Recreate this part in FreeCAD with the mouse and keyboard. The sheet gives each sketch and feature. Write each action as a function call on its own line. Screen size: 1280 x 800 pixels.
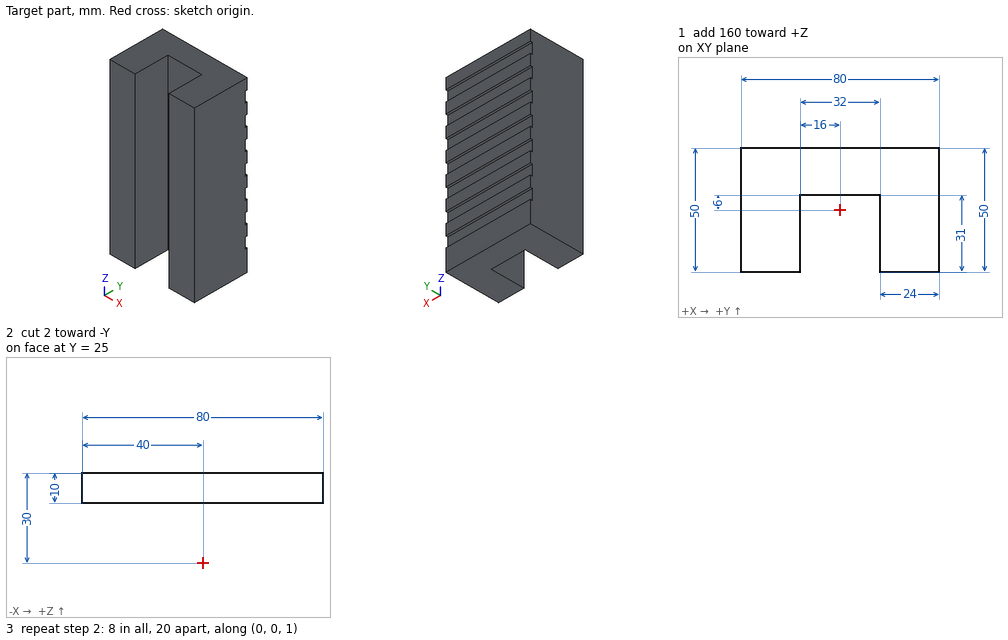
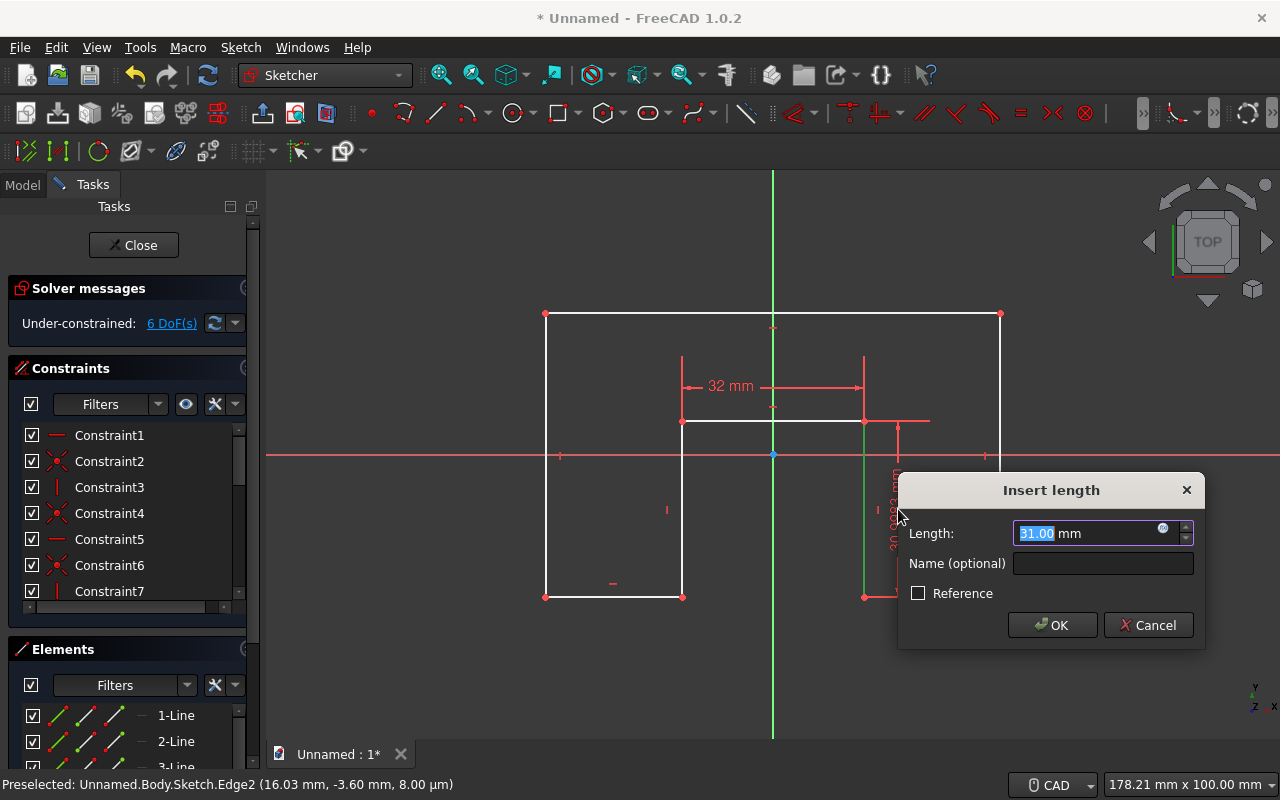
text(31)
key(Return)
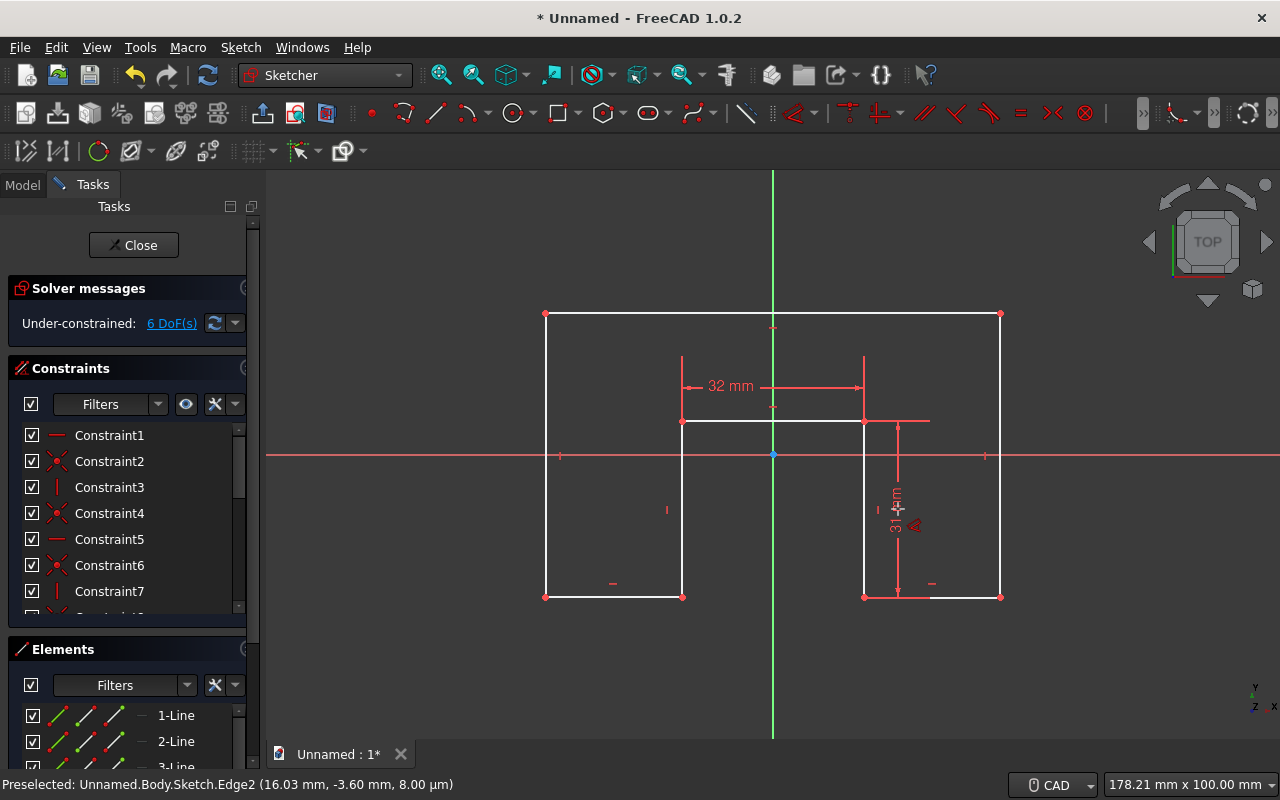
click(905, 598)
click(932, 632)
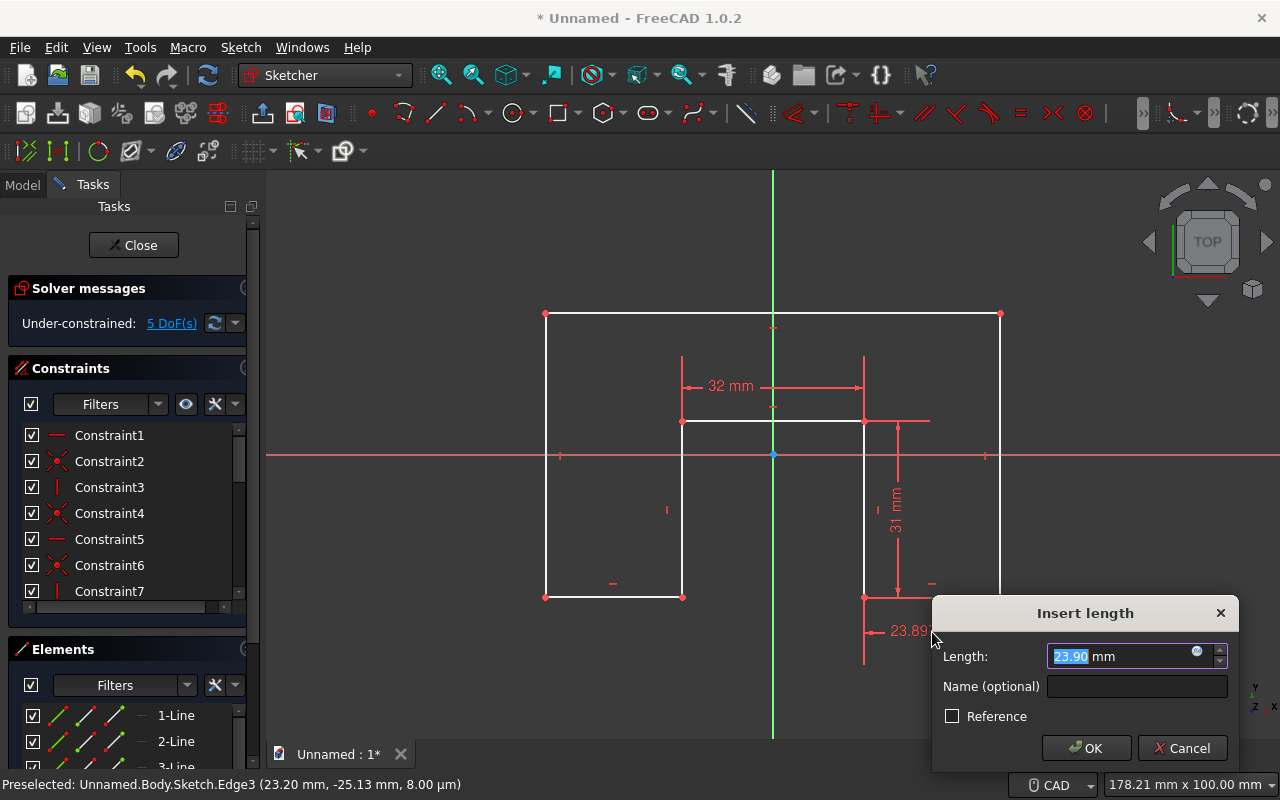
text(24)
key(Return)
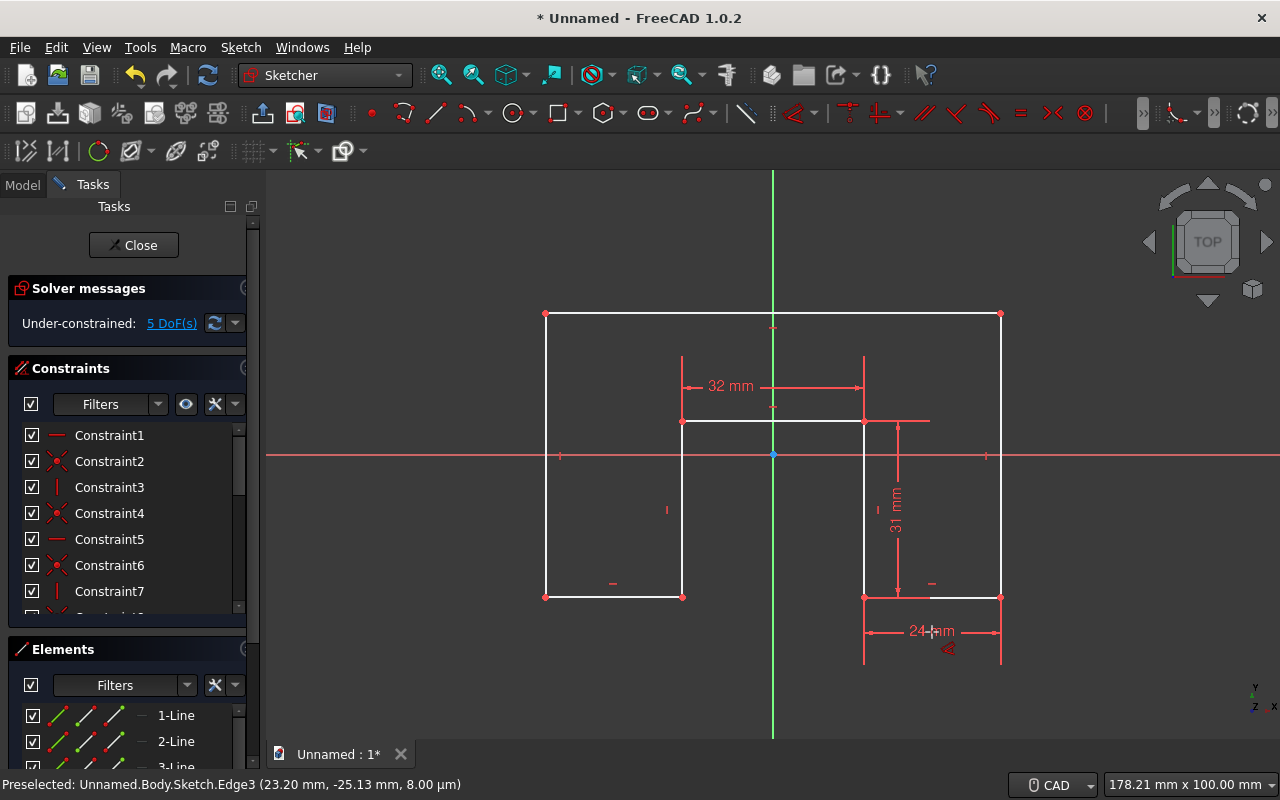
click(1001, 512)
click(1035, 390)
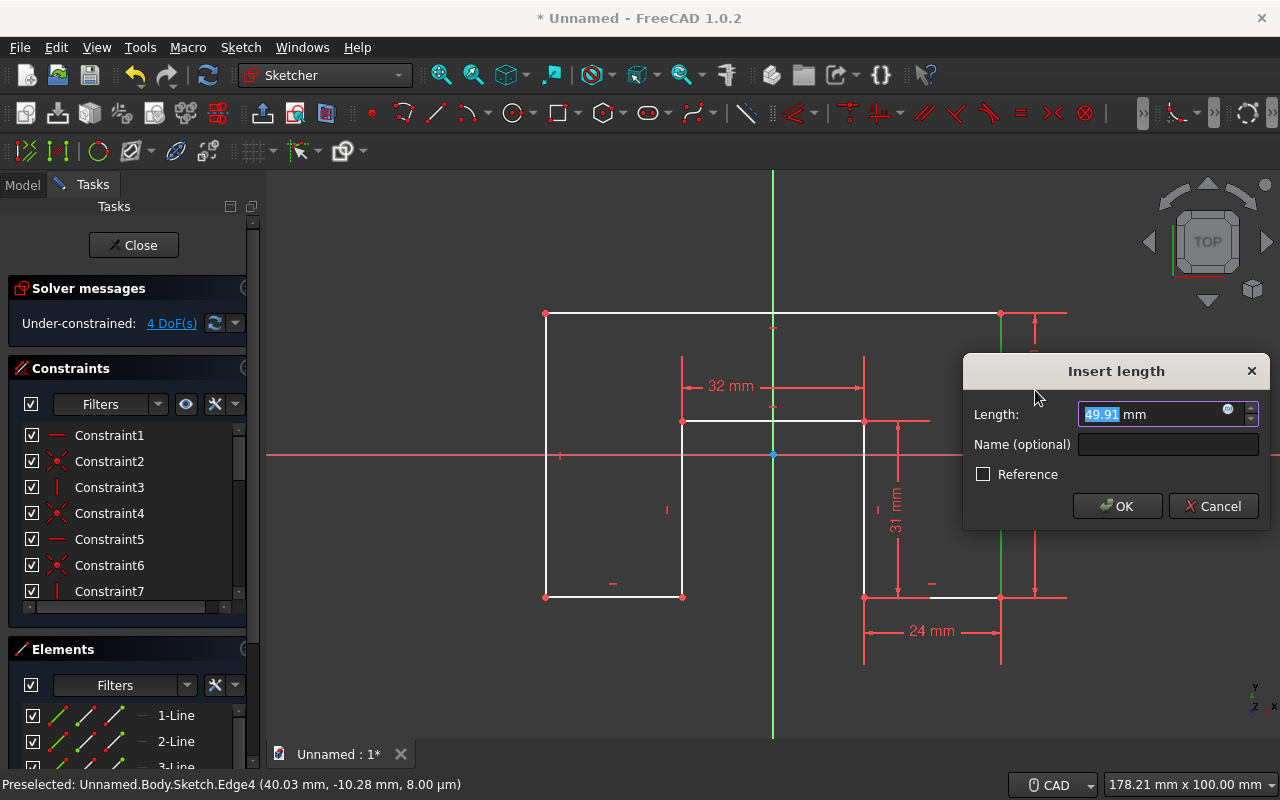
text(50)
key(Return)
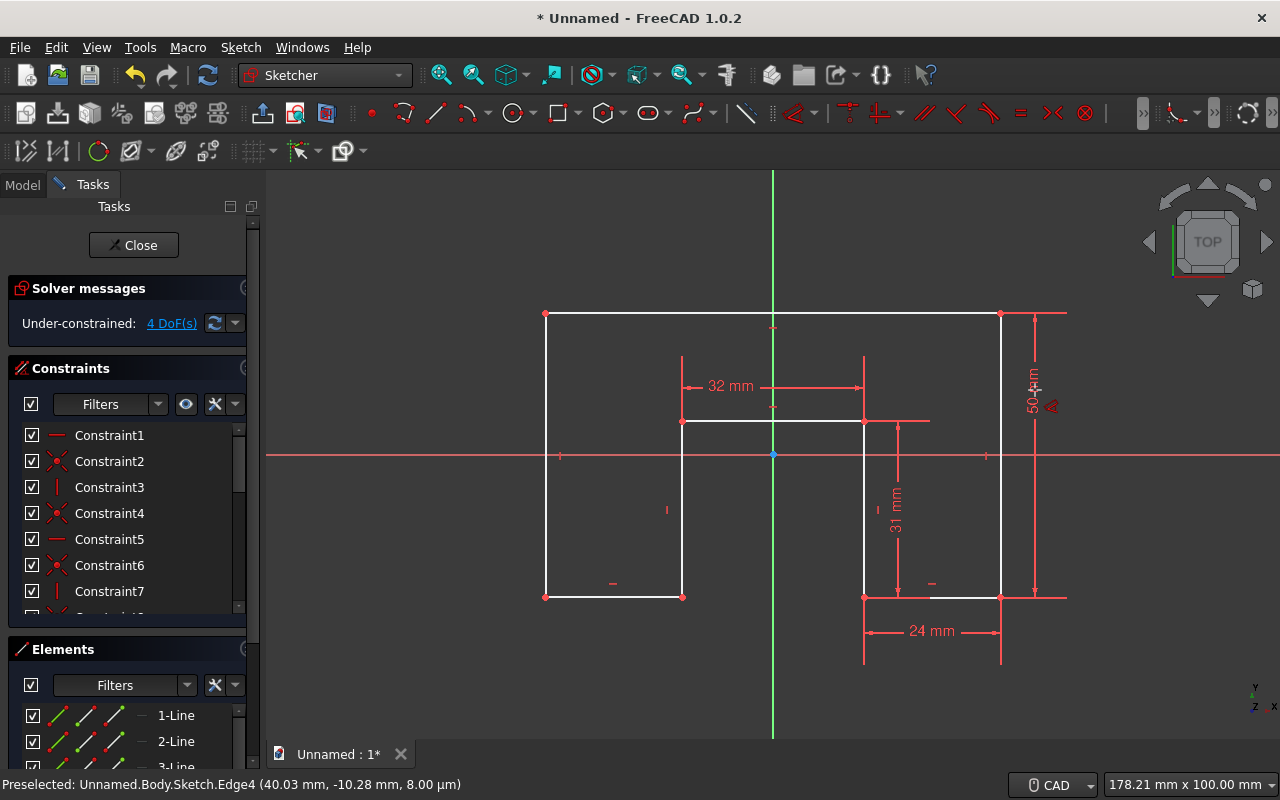
click(864, 313)
click(669, 279)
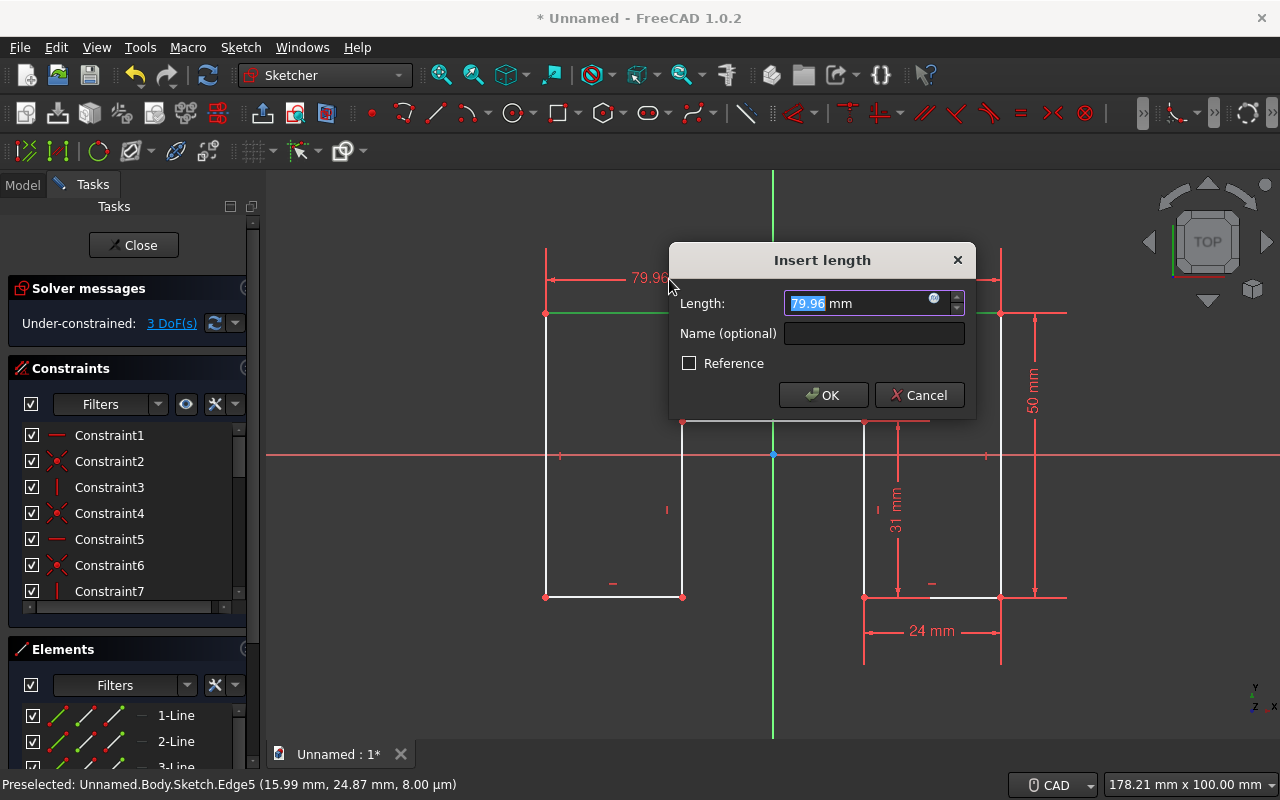
text(80)
key(Return)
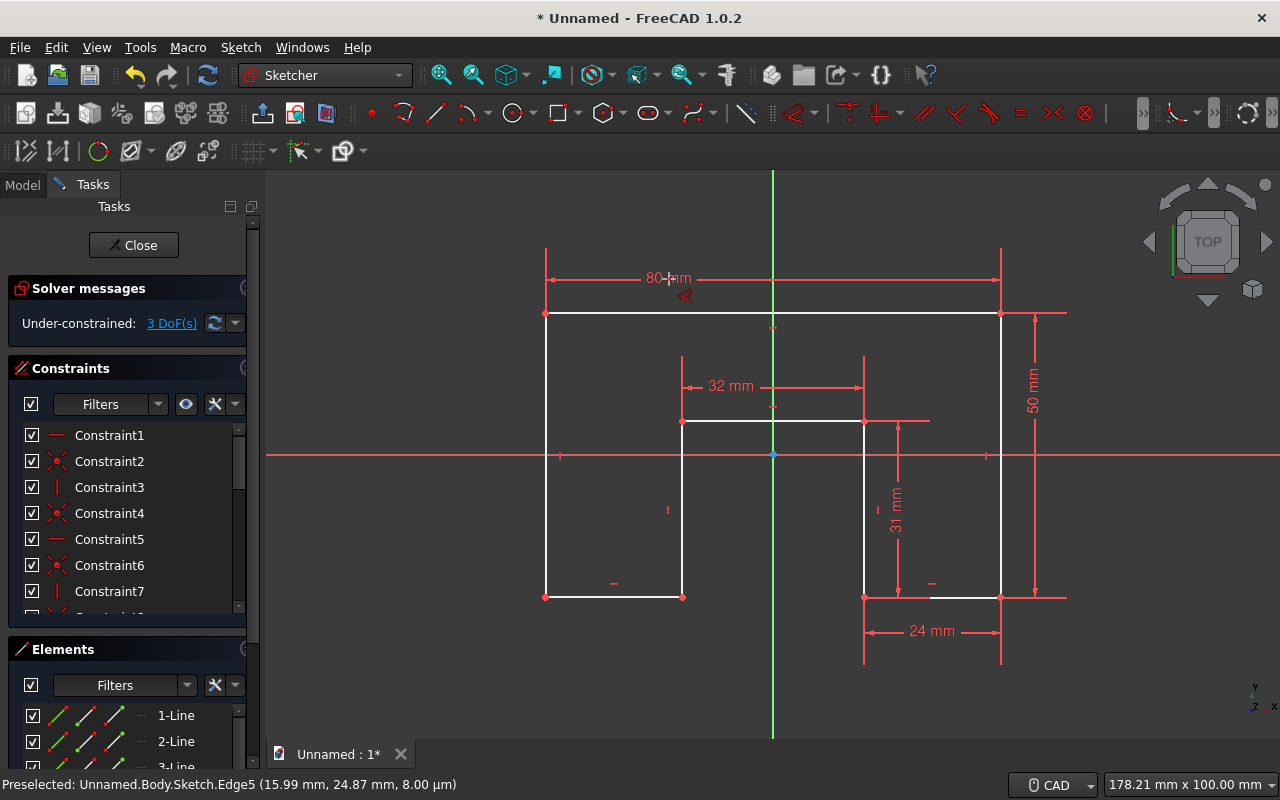
click(546, 398)
click(512, 390)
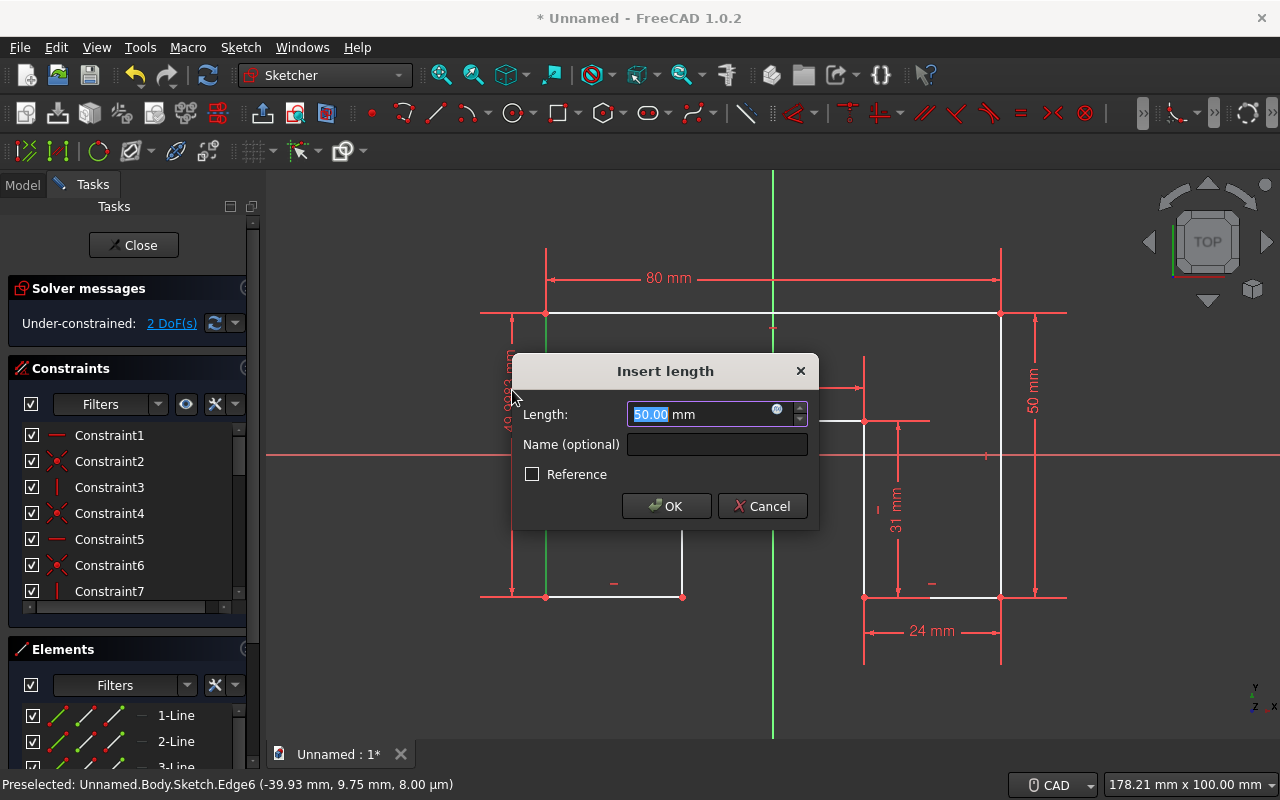
text(50)
key(Return)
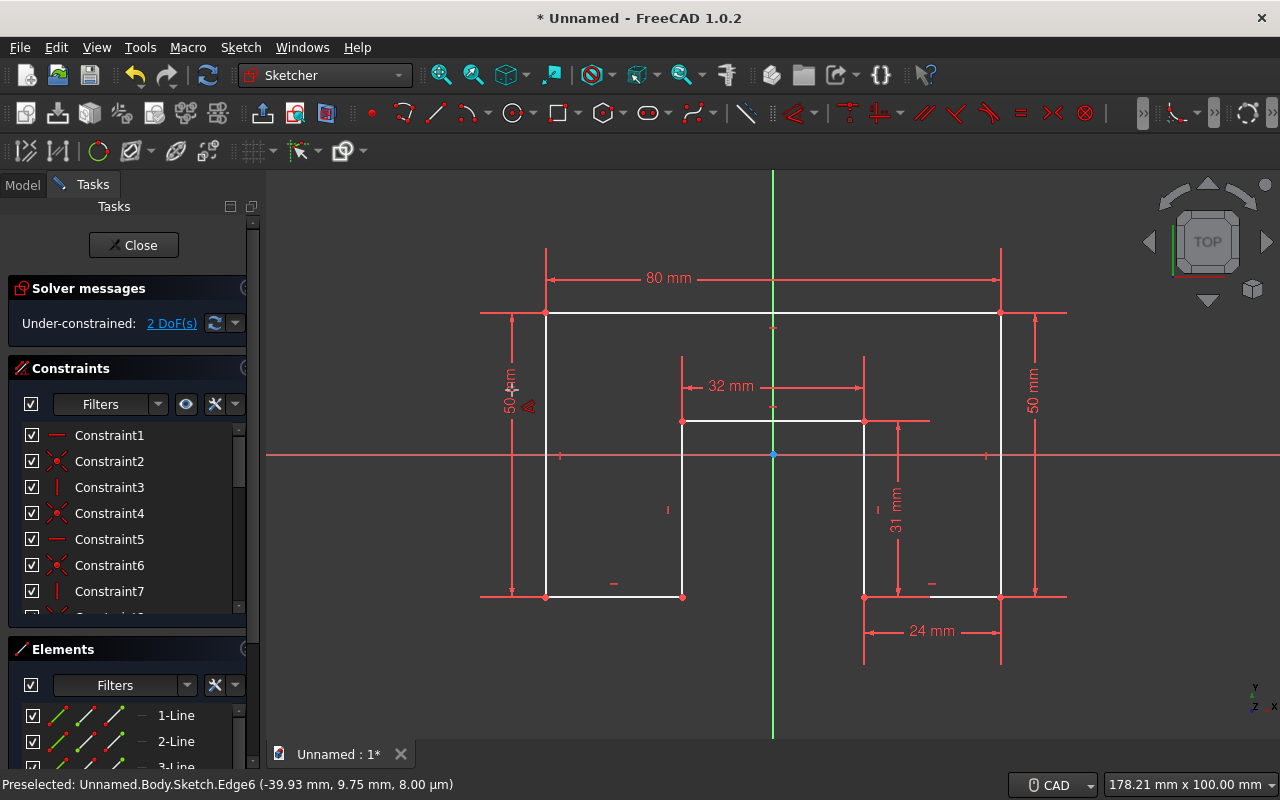
click(682, 421)
click(648, 438)